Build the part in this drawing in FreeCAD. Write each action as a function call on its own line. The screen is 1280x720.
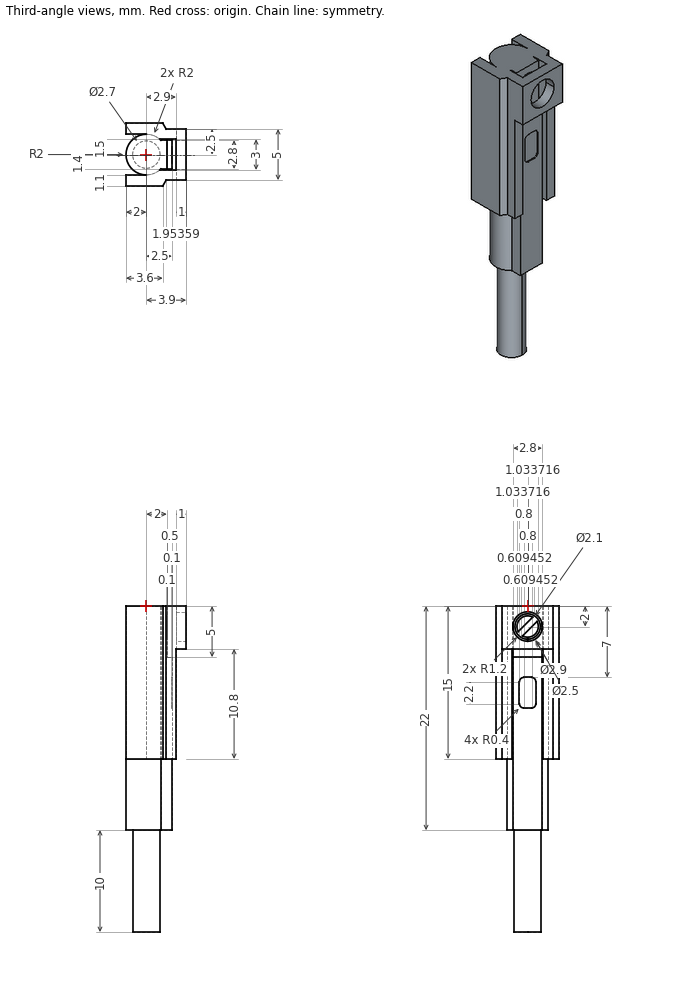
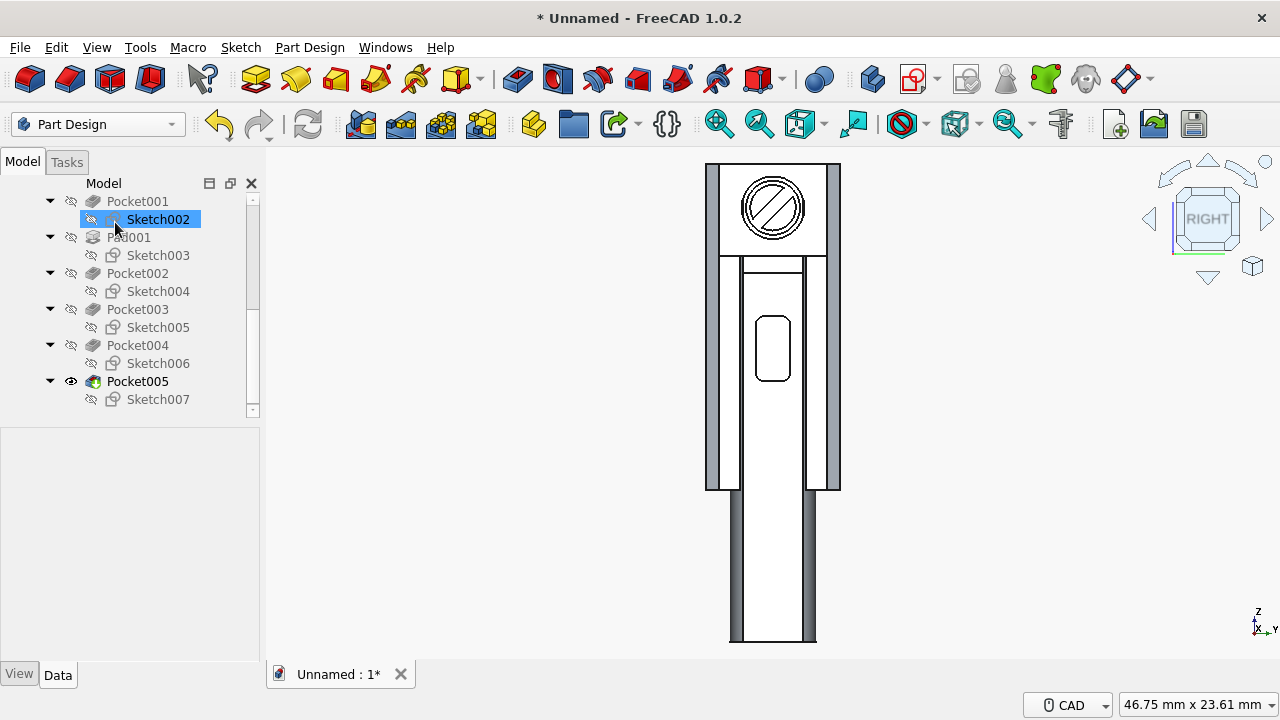
key(5)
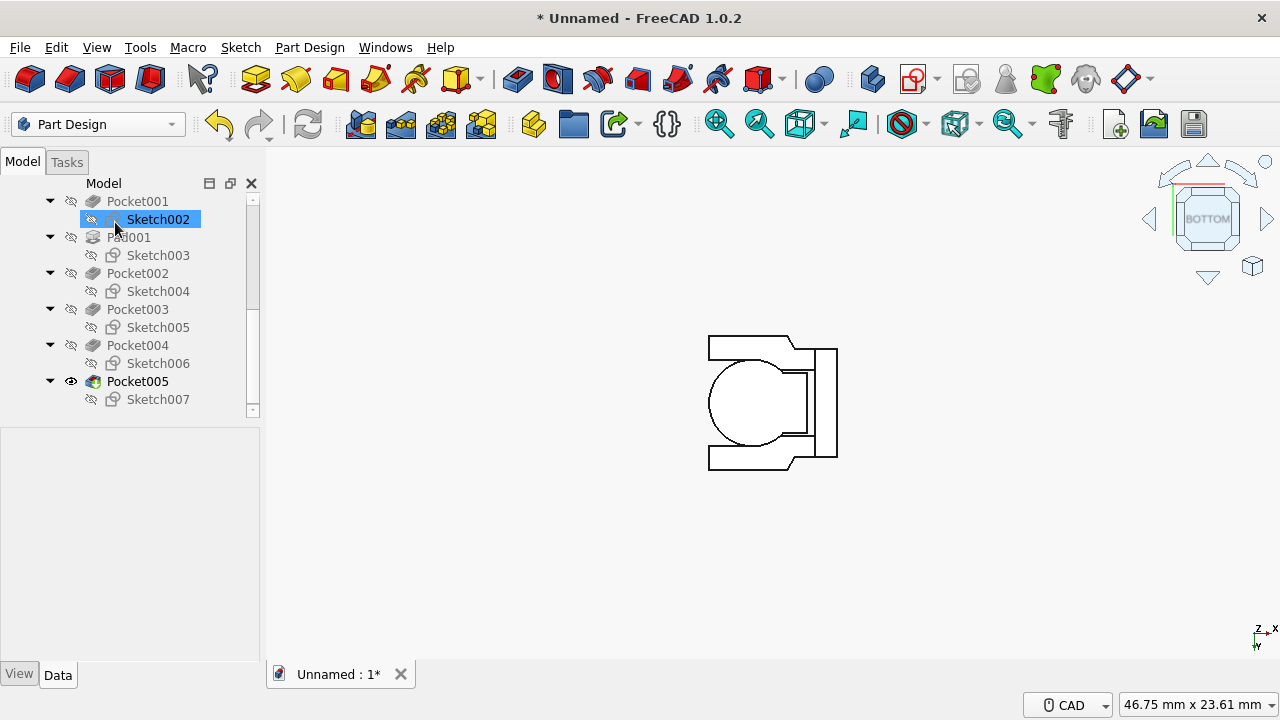
click(720, 124)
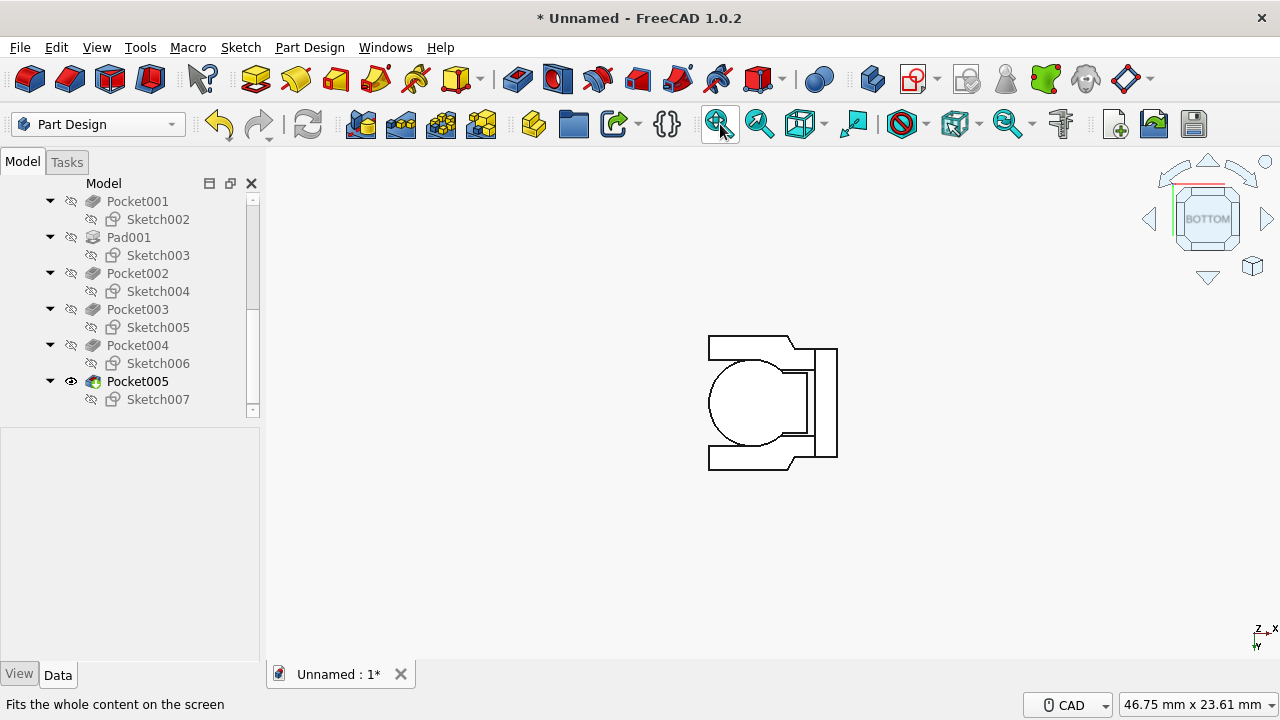
click(758, 402)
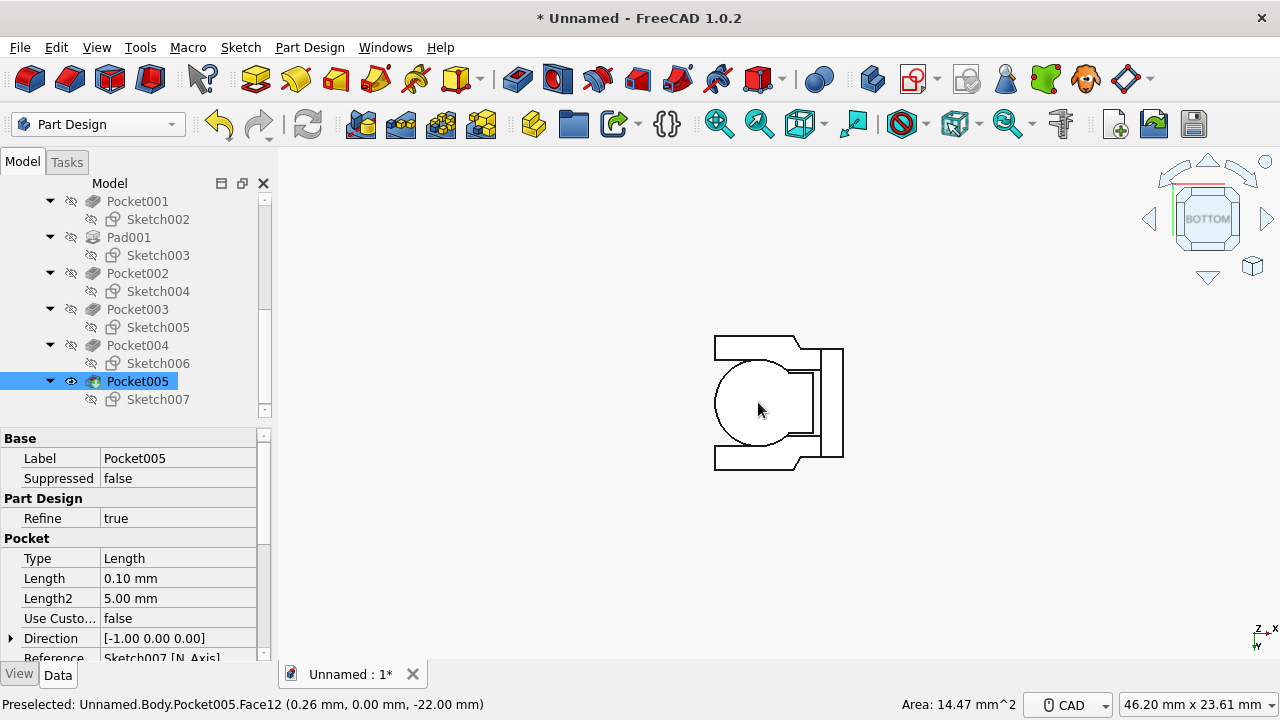
click(914, 80)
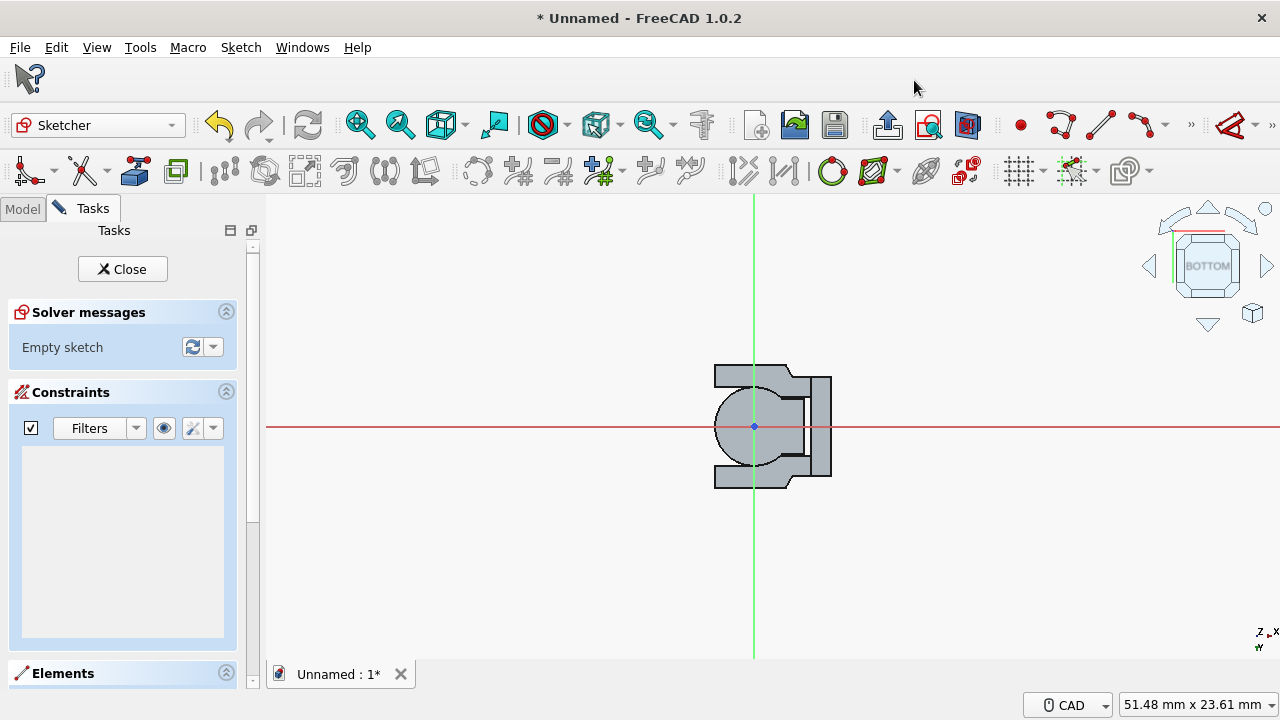
scroll(767, 426, up, 8)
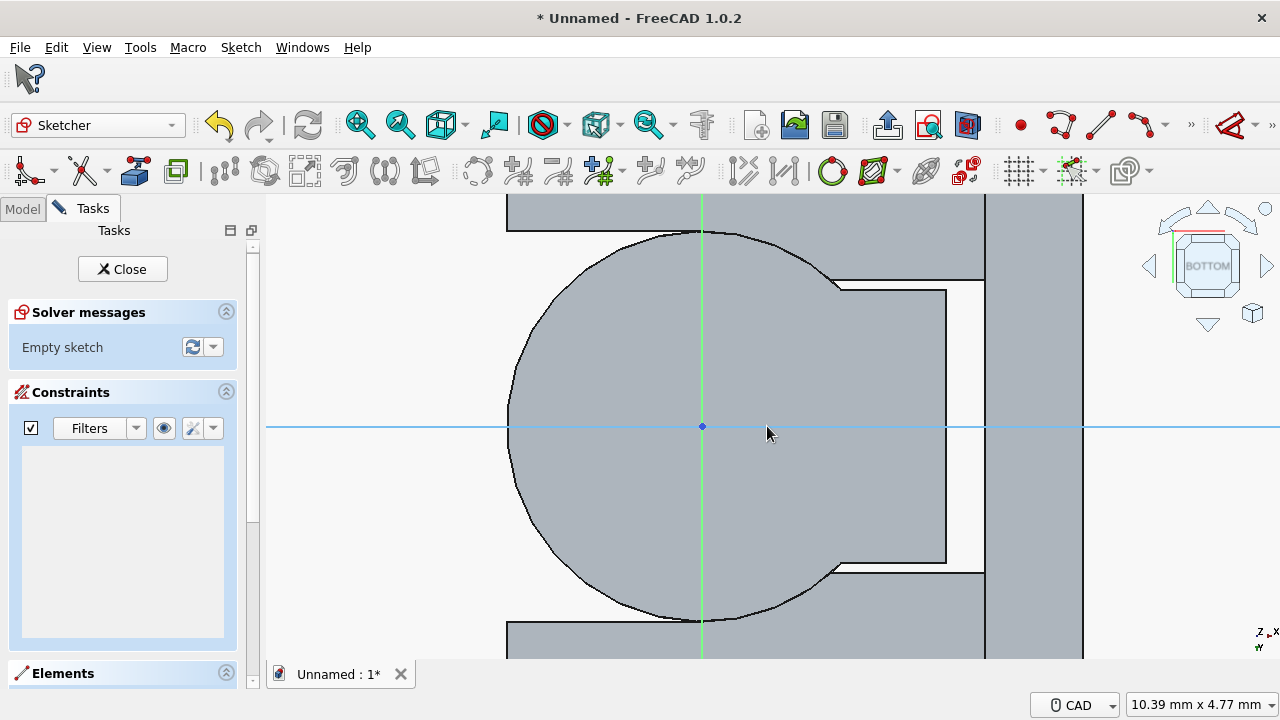
key(g)
key(c)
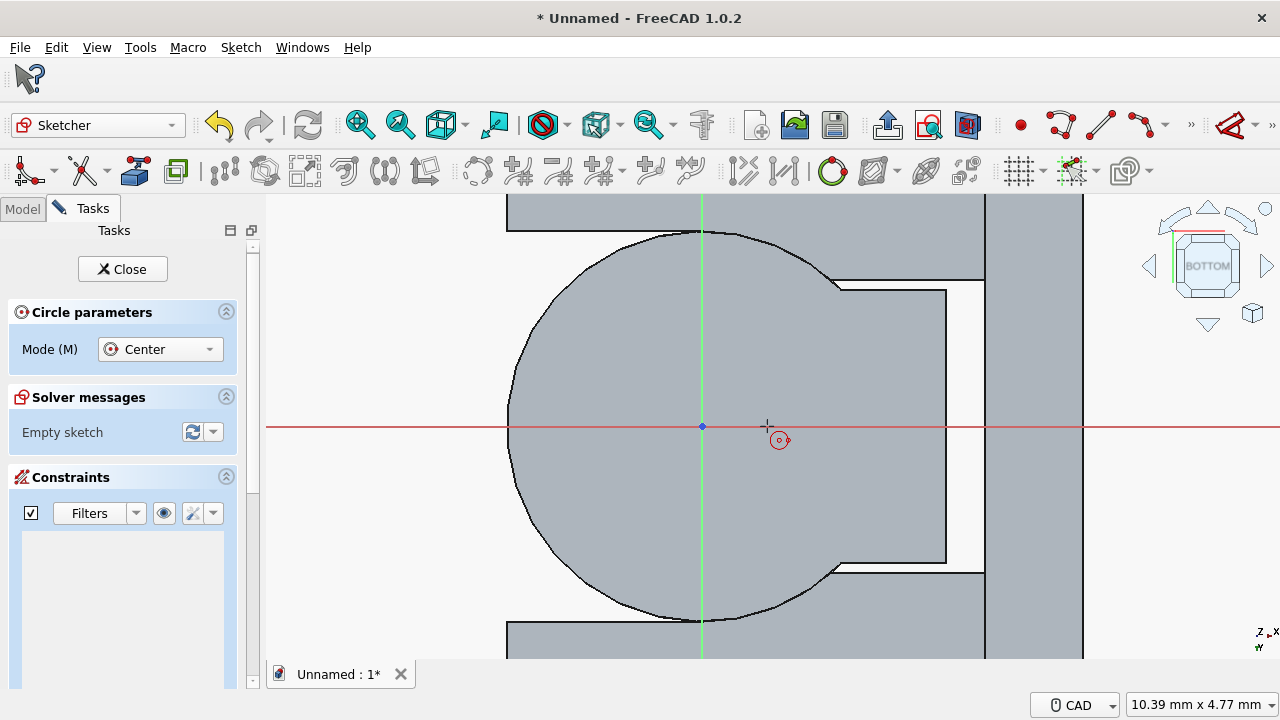
click(702, 426)
click(795, 333)
key(Escape)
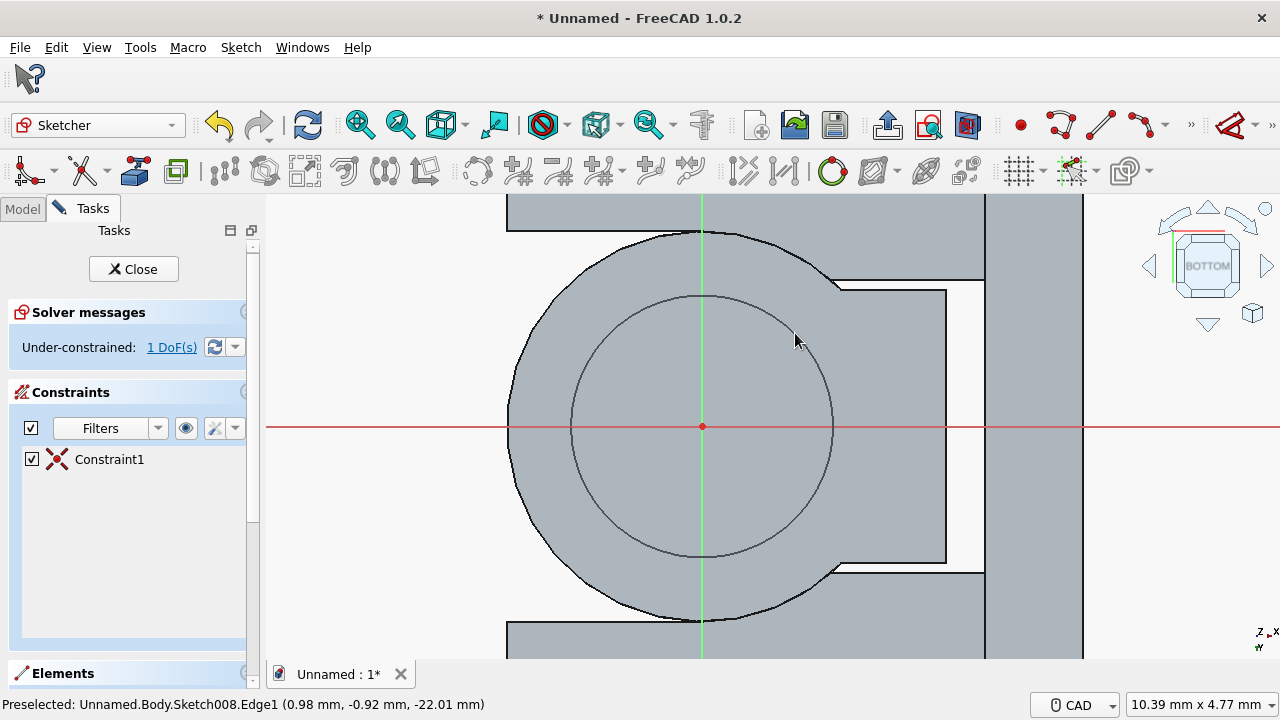
click(1230, 126)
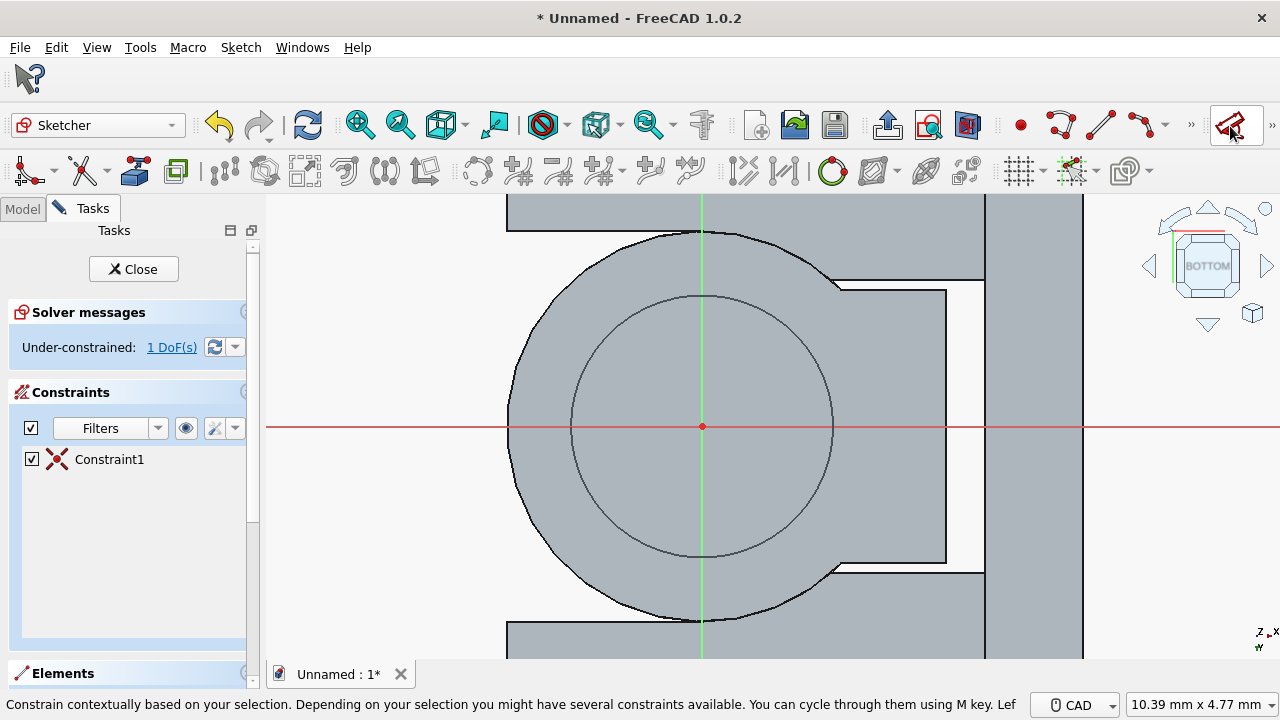
click(795, 334)
click(818, 311)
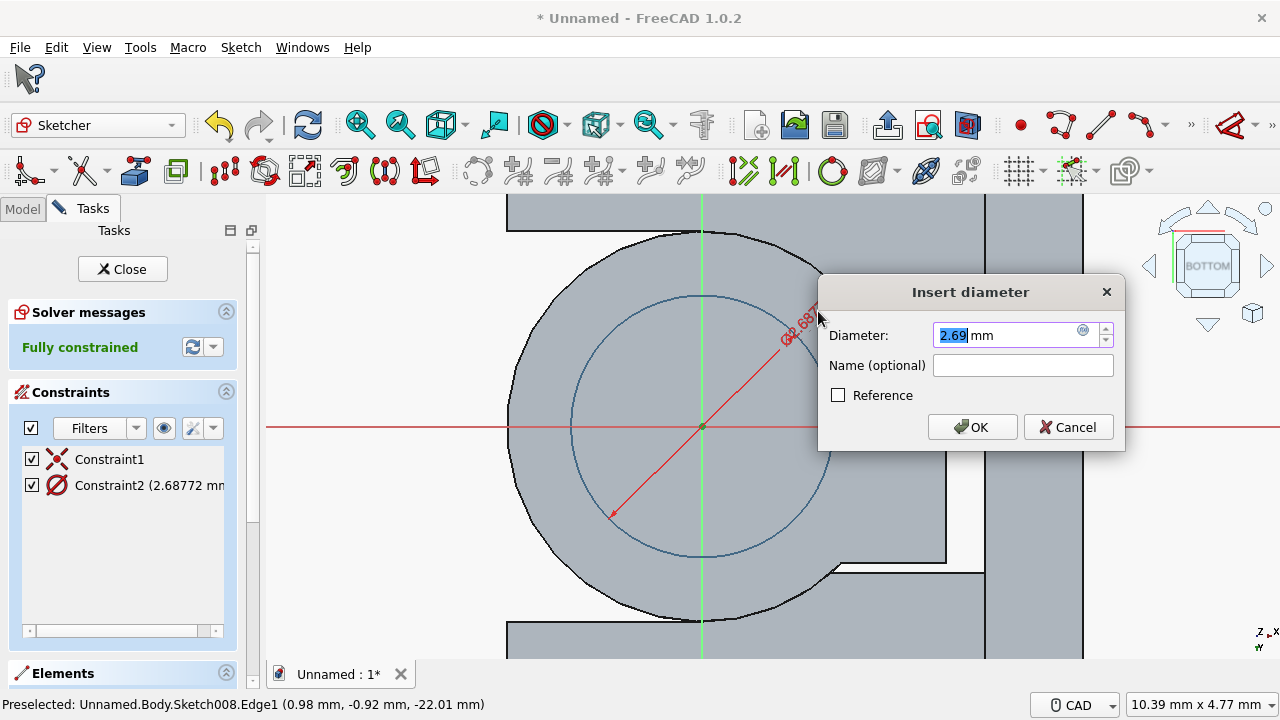
text(2.7)
key(Return)
key(Escape)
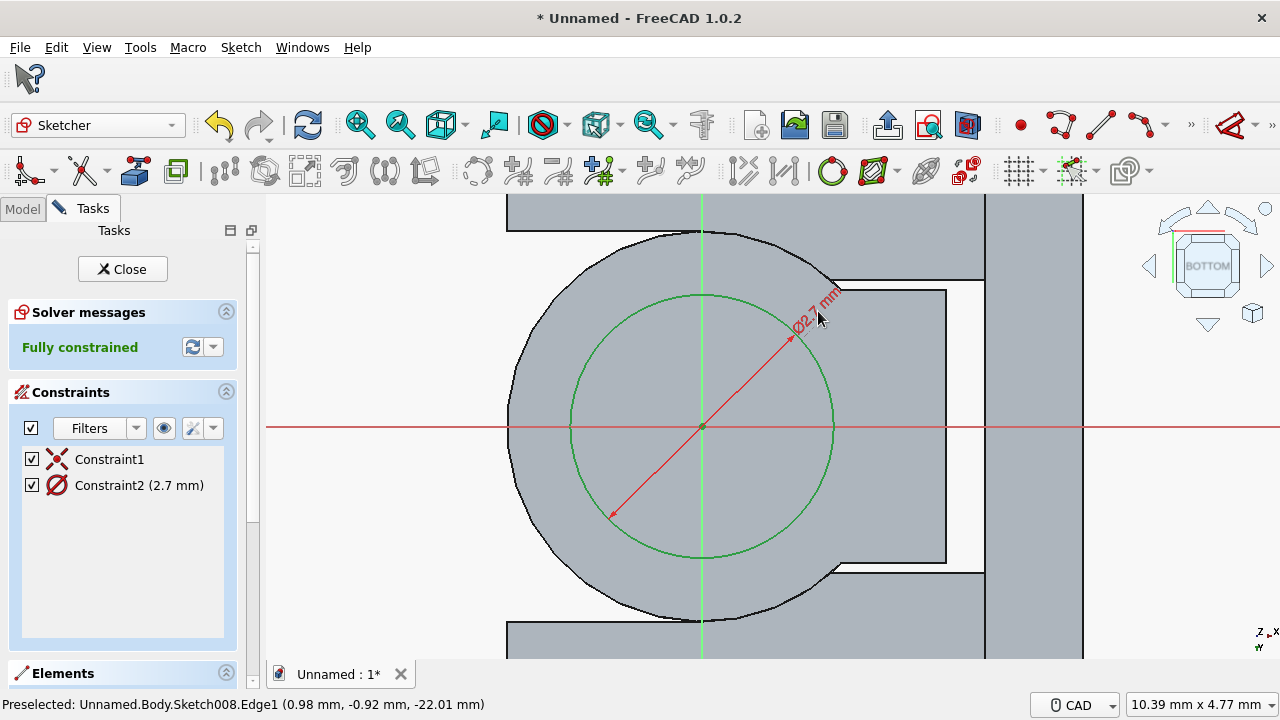
click(123, 269)